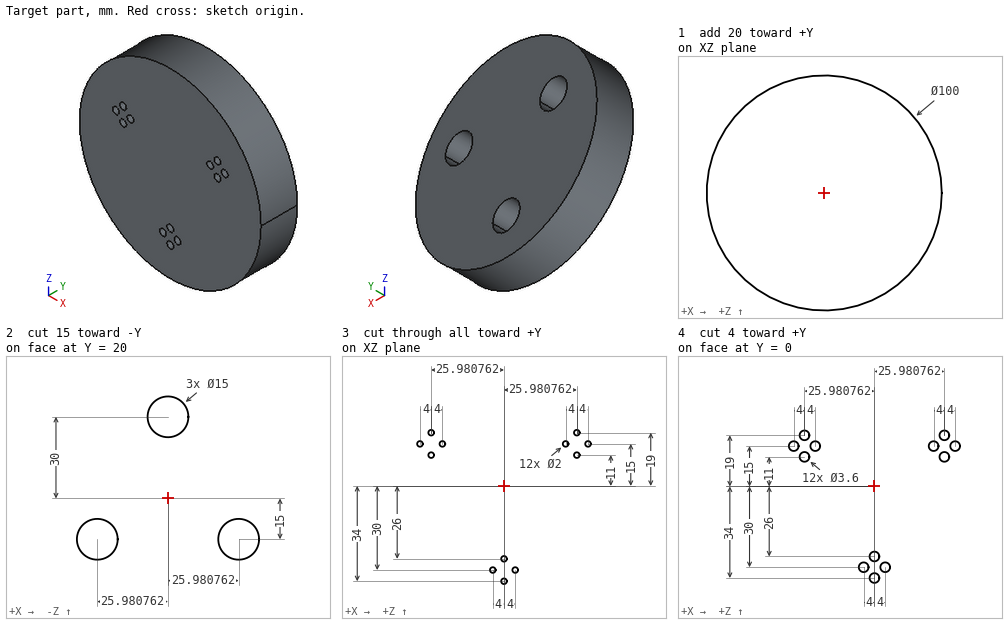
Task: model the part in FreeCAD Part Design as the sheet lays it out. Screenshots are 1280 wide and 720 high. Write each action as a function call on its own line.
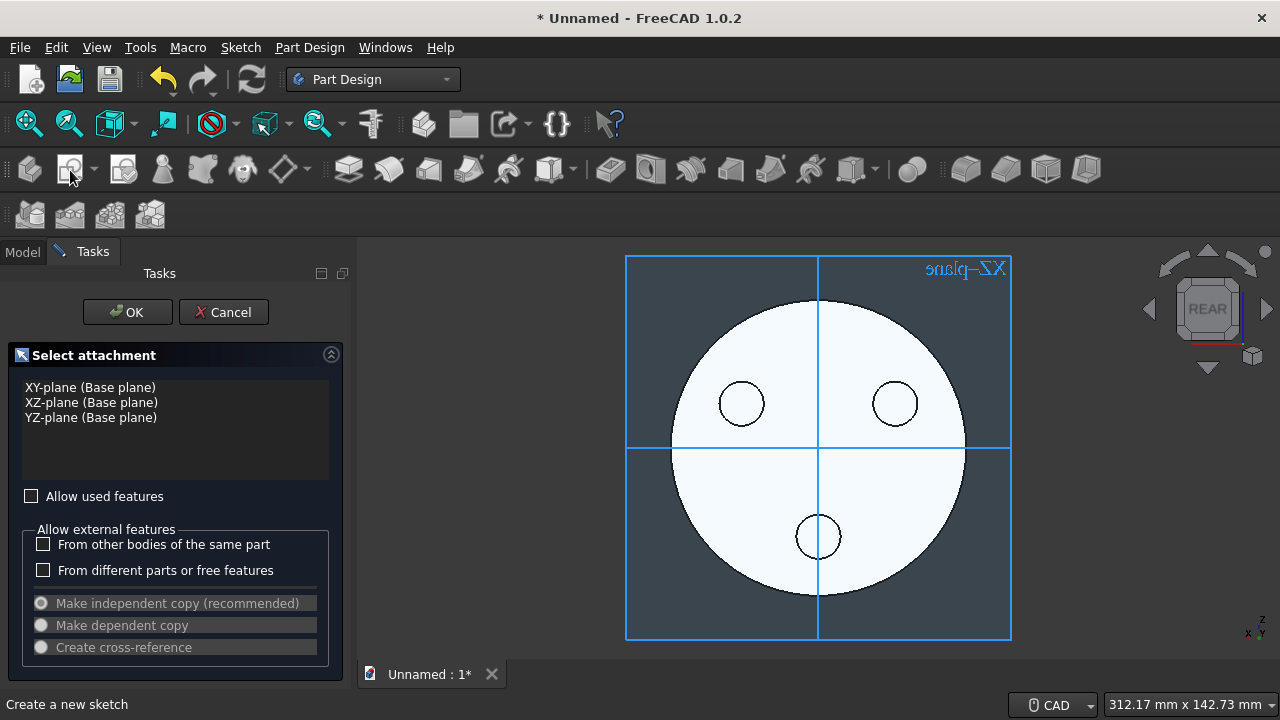
click(82, 402)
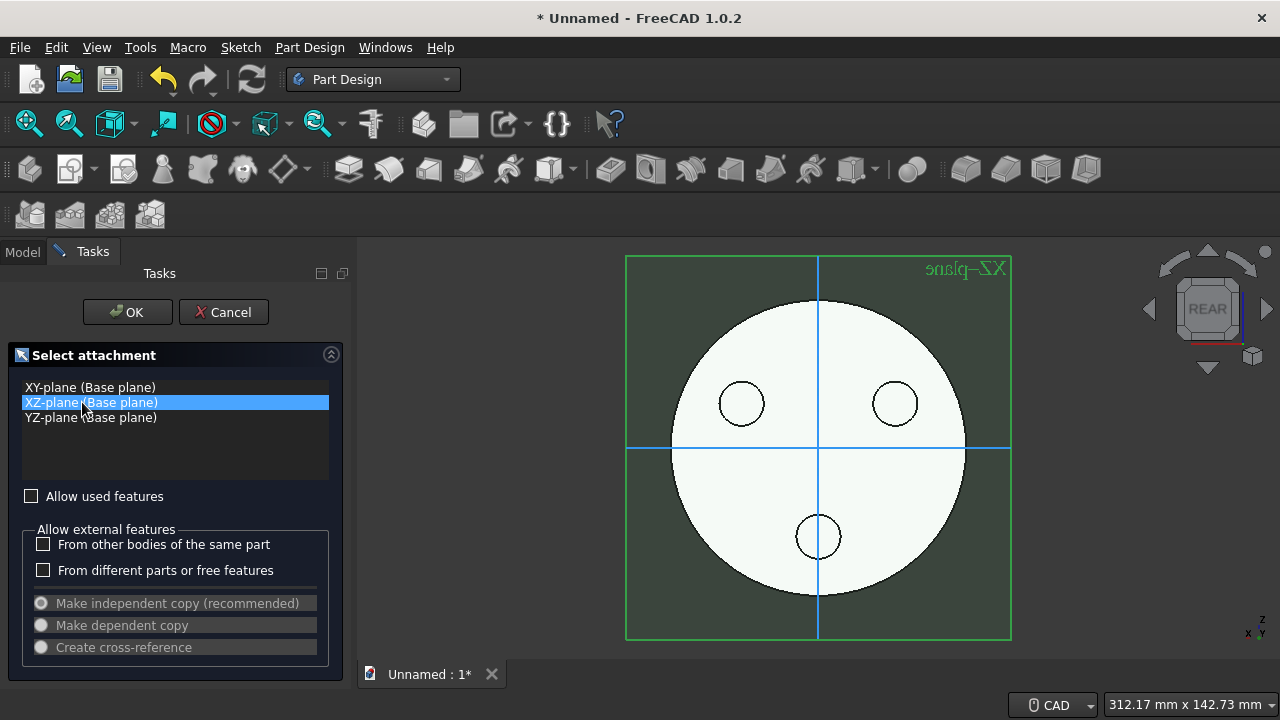
click(128, 312)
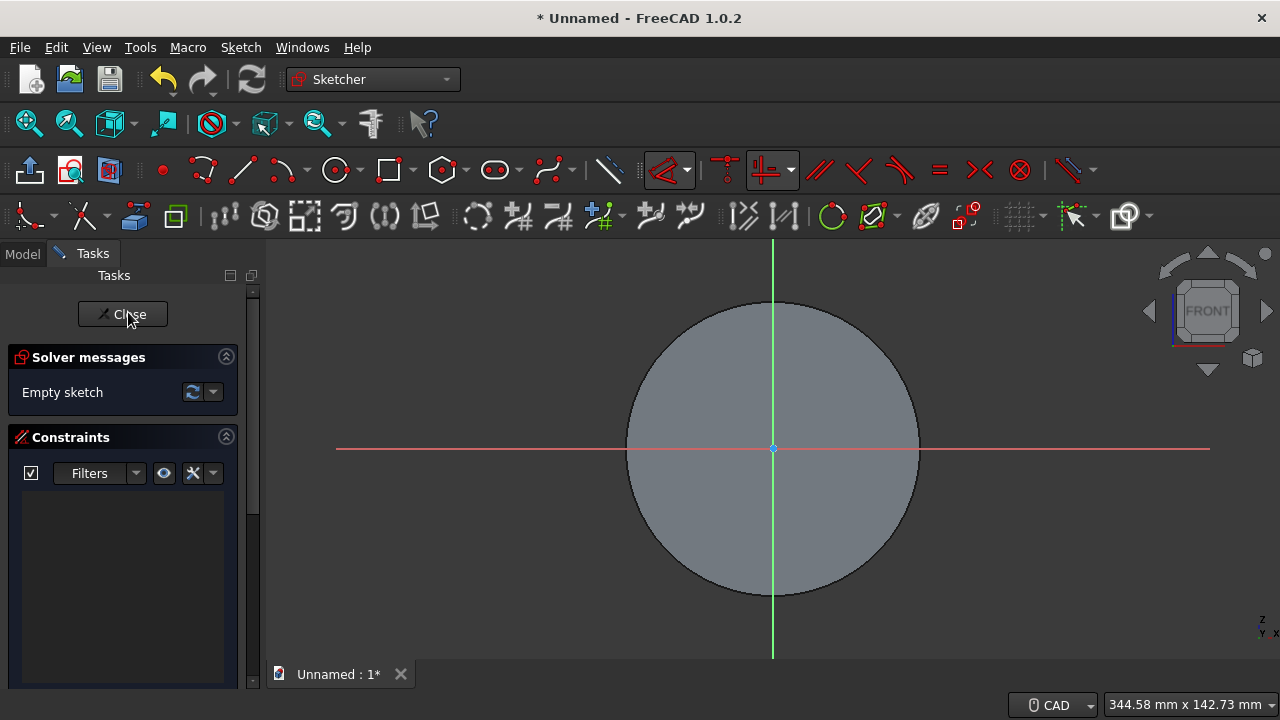
scroll(912, 516, up, 2)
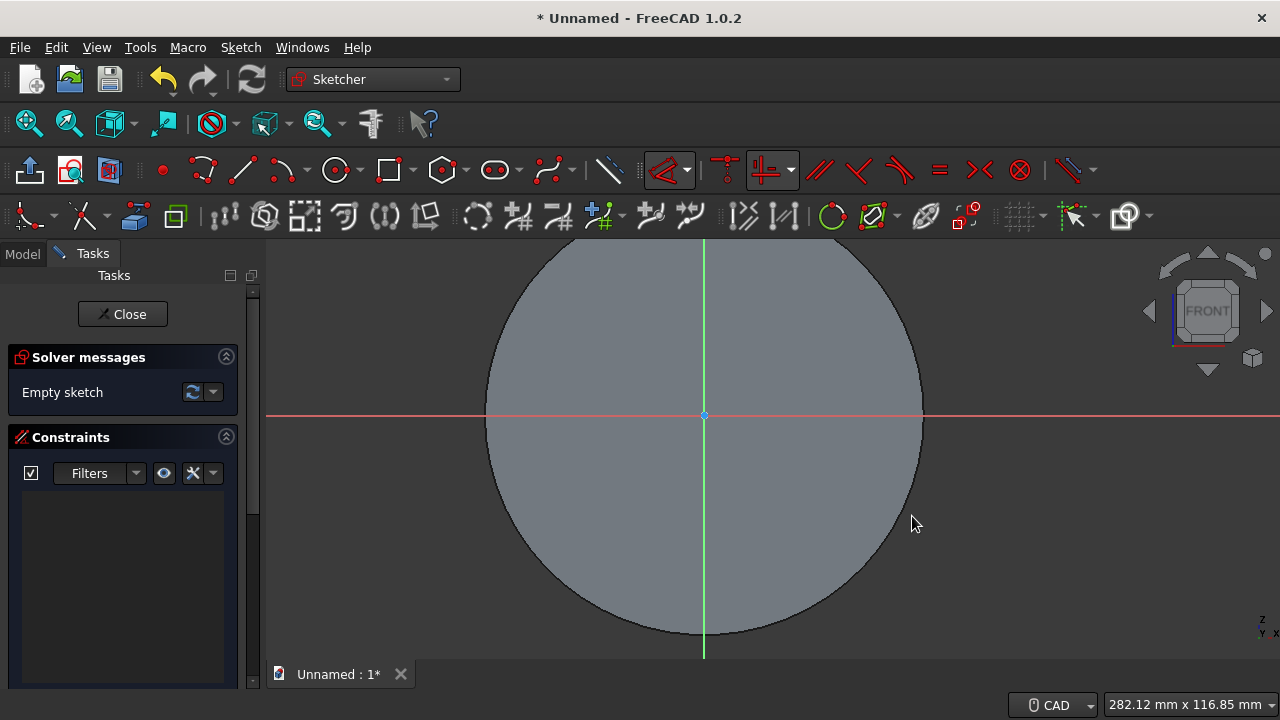
click(336, 170)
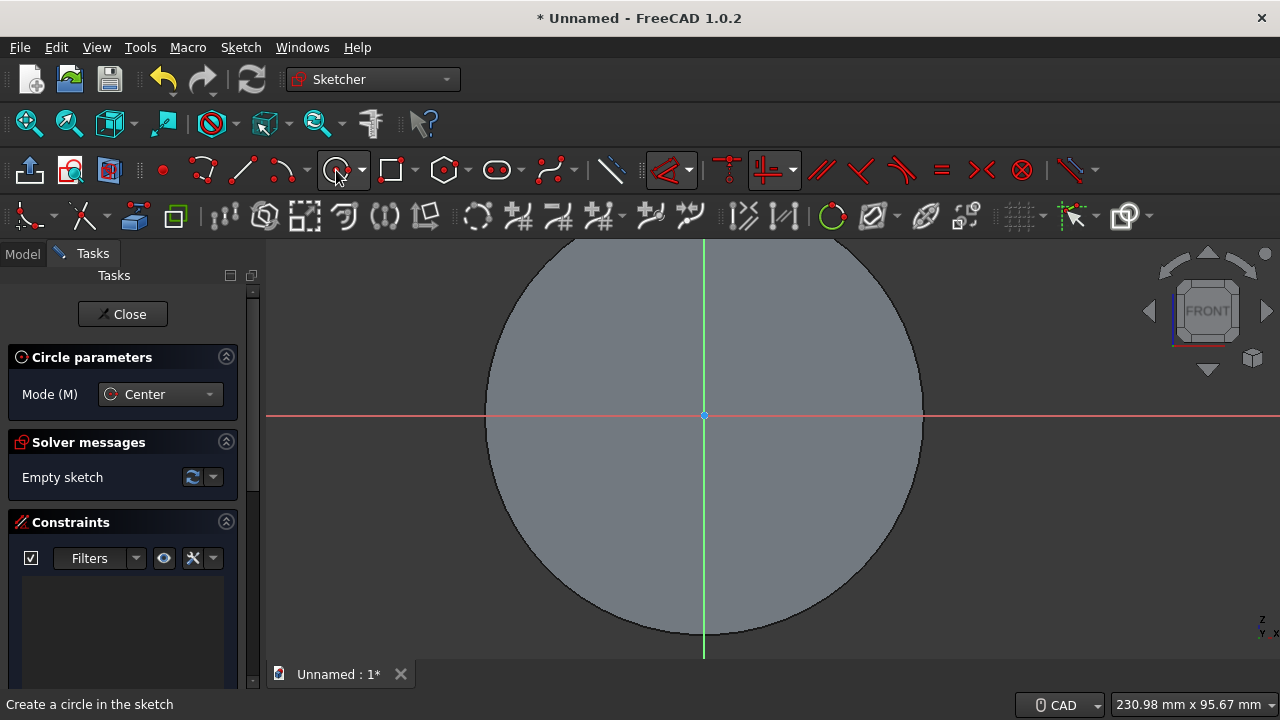
scroll(818, 332, up, 9)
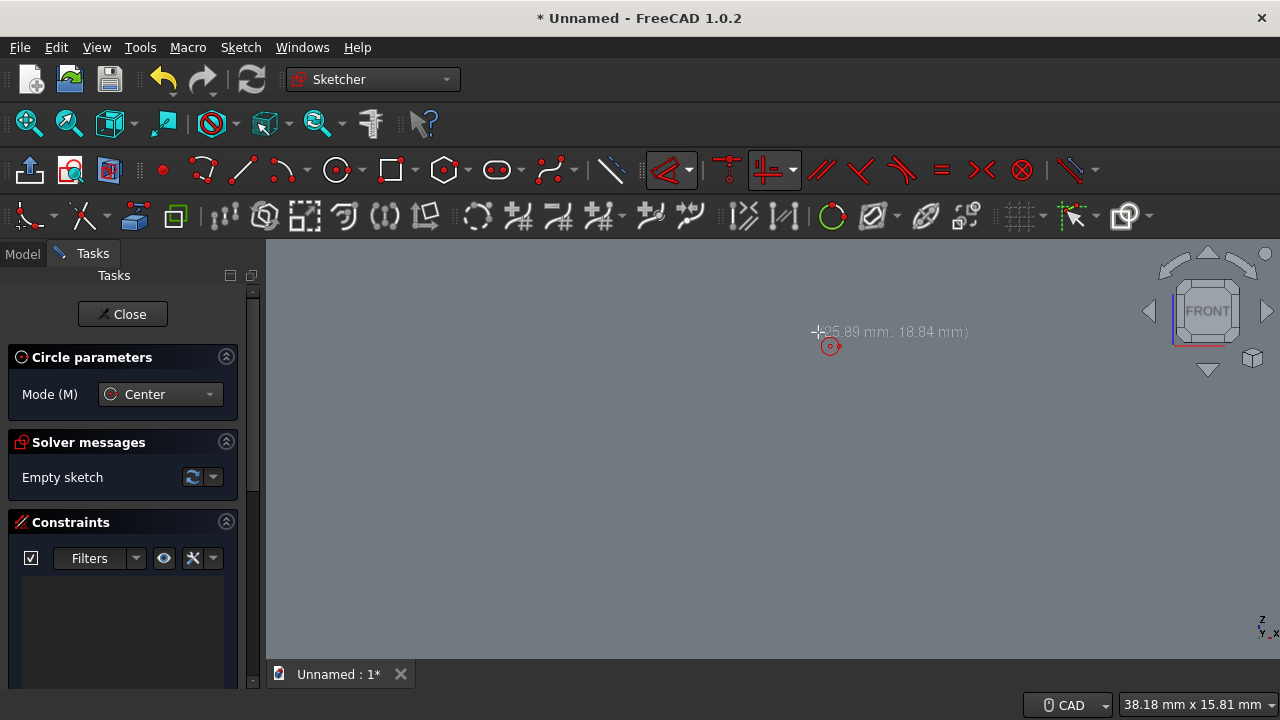
scroll(819, 333, down, 9)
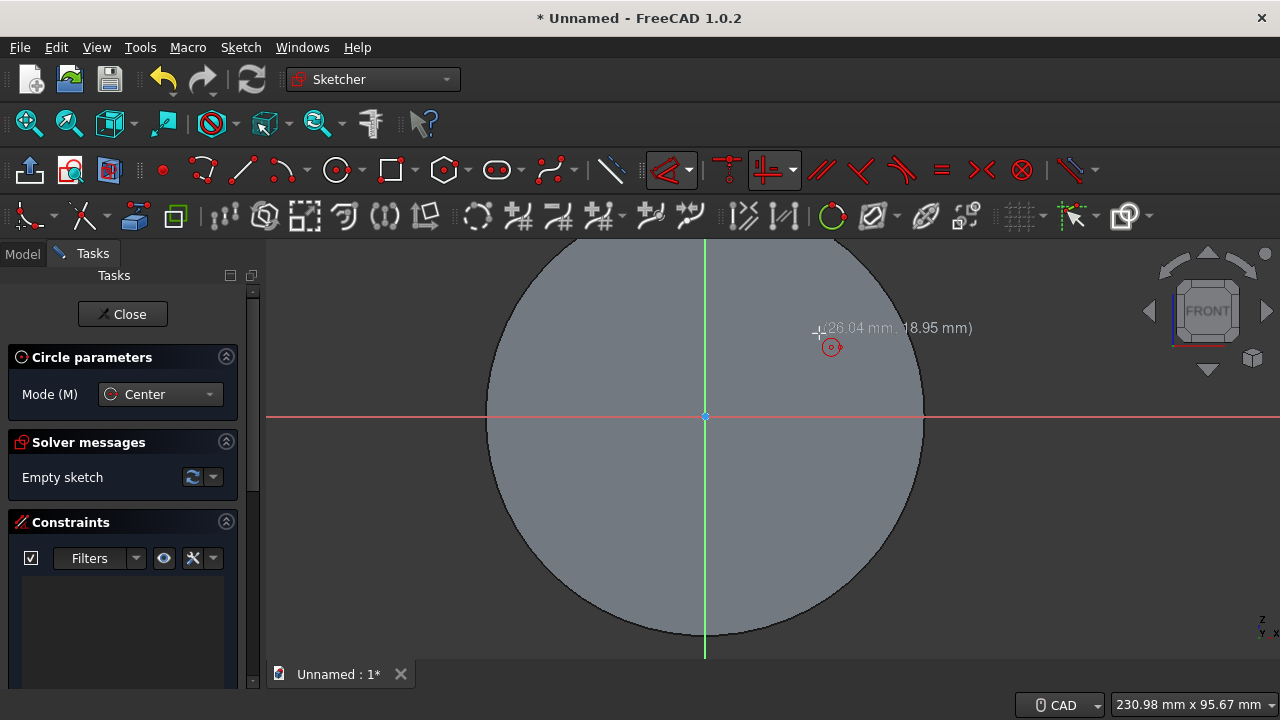
click(819, 333)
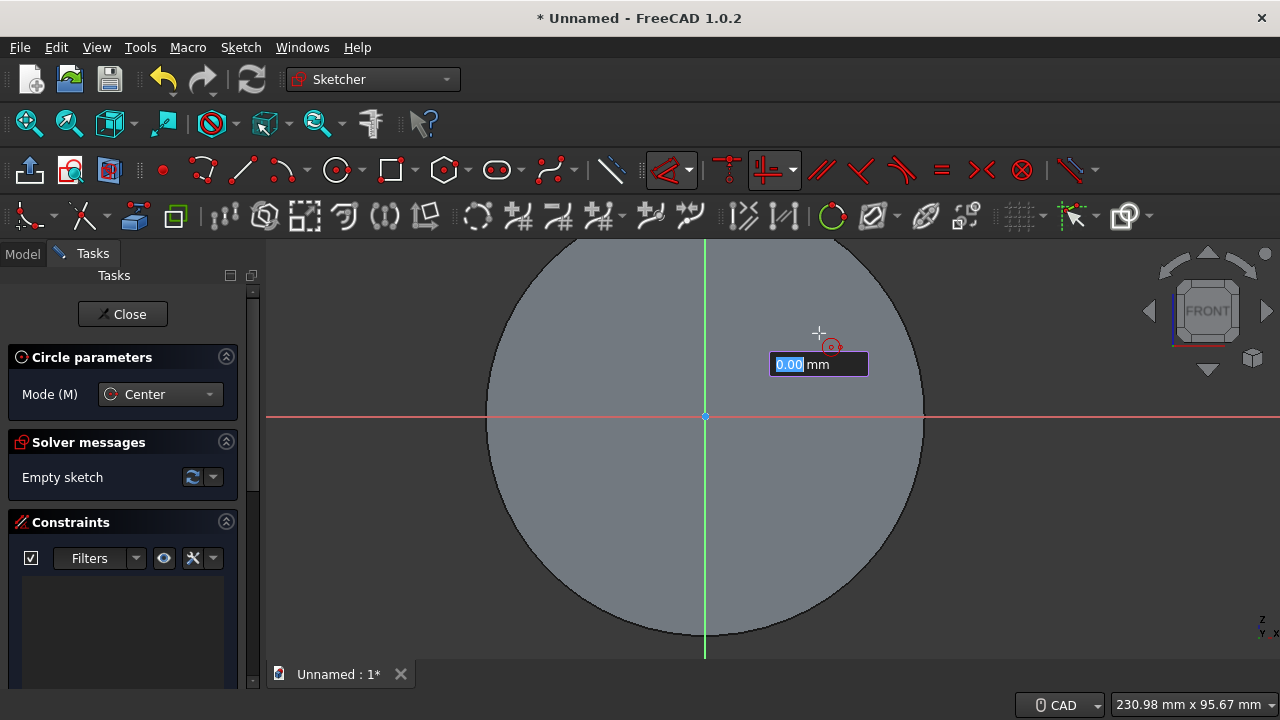
scroll(822, 330, up, 7)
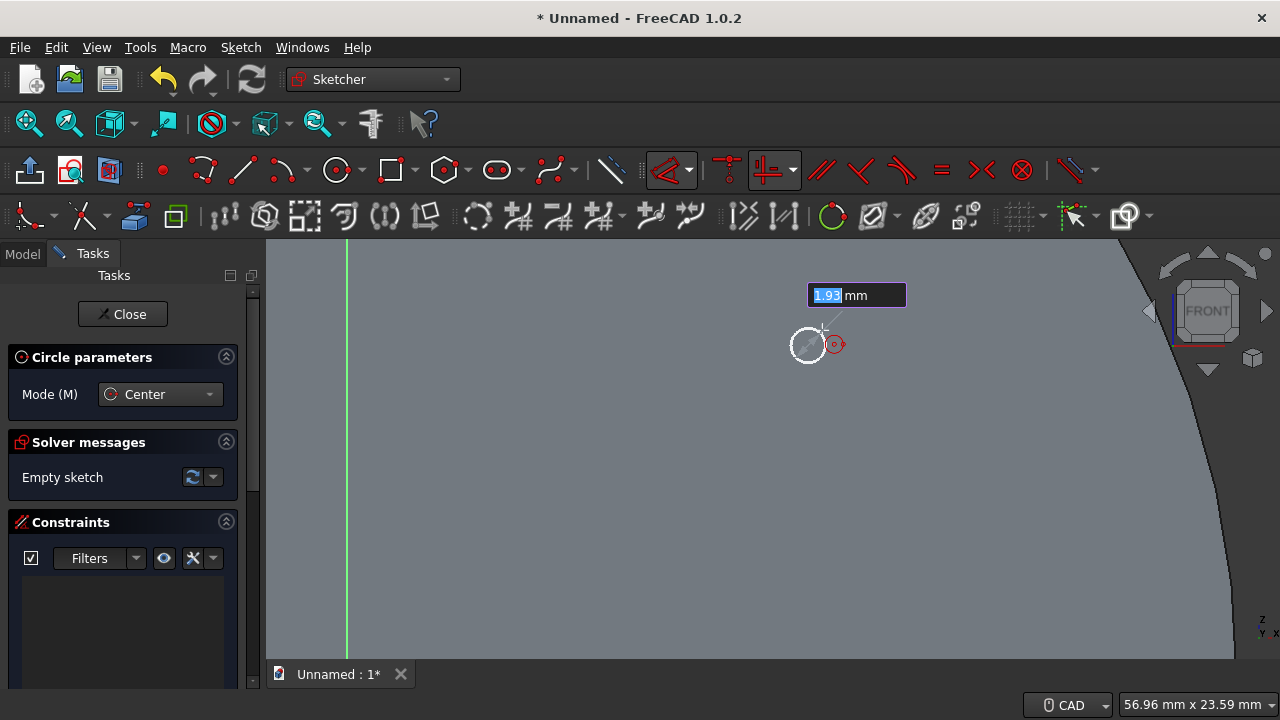
click(822, 330)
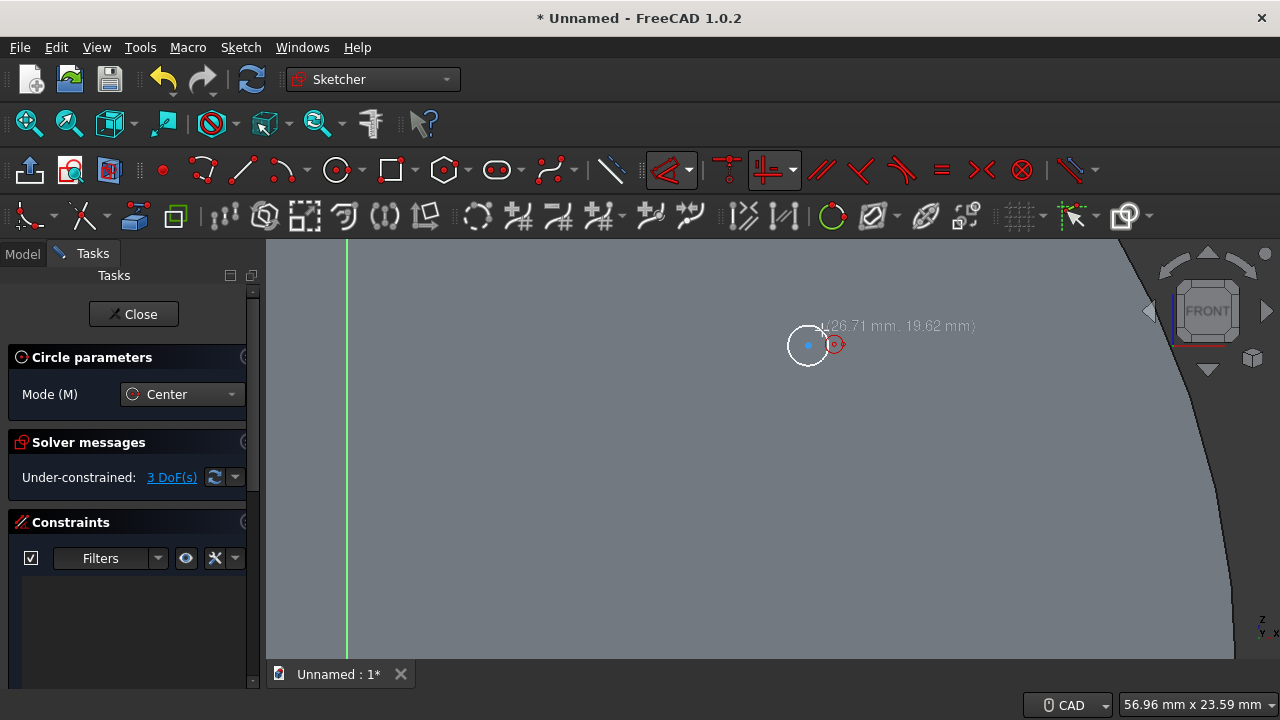
scroll(880, 413, up, 2)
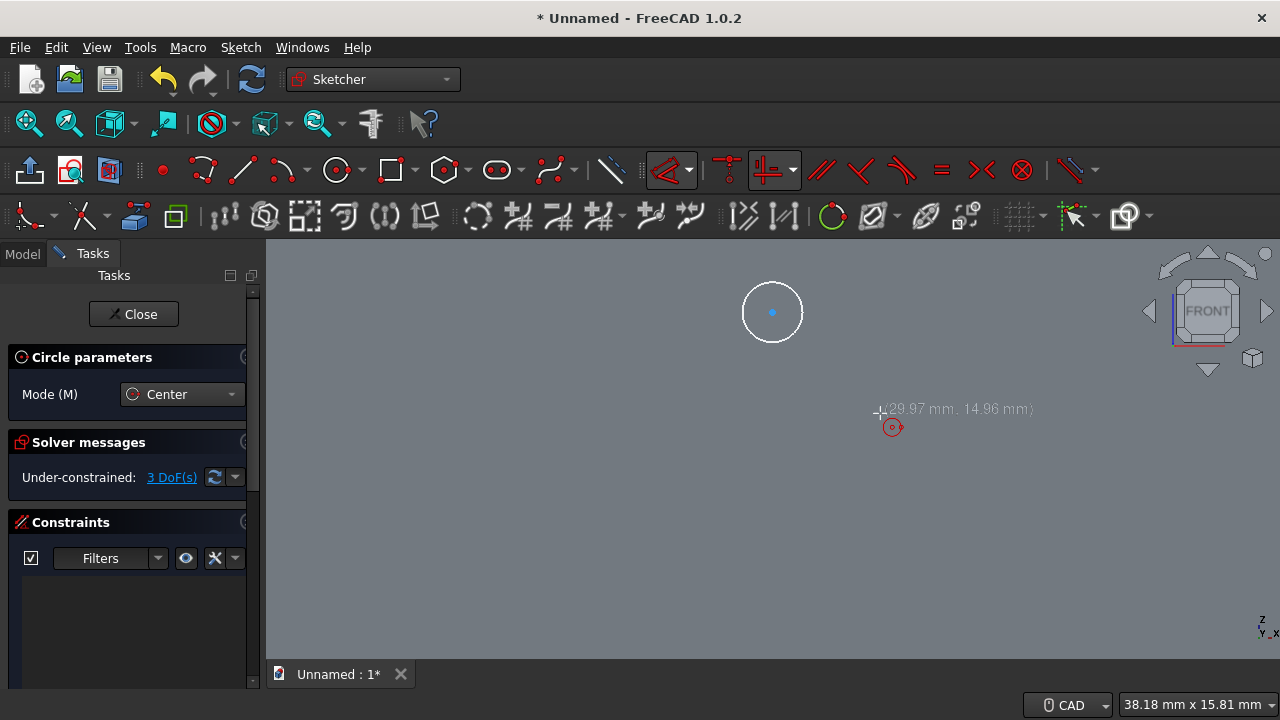
scroll(827, 338, down, 9)